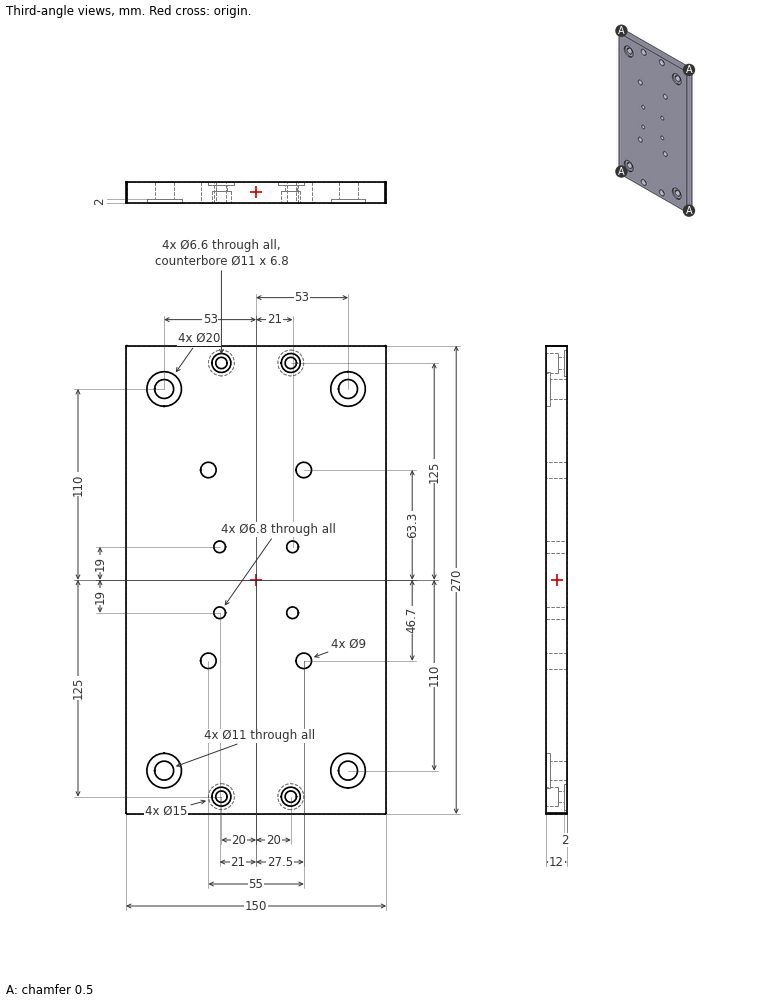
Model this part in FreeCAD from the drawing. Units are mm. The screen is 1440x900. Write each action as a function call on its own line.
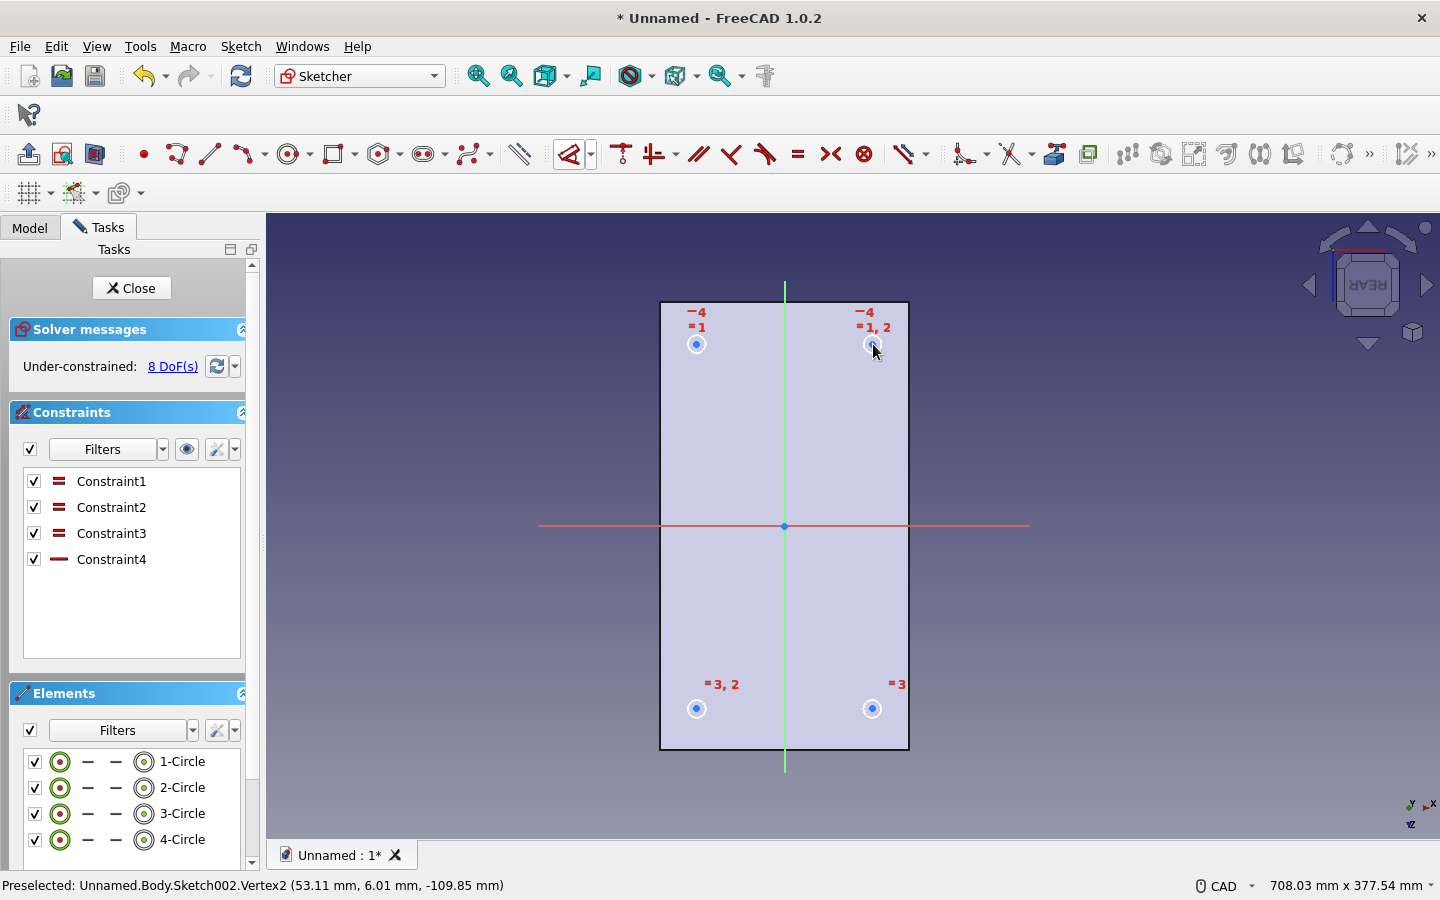
click(697, 344)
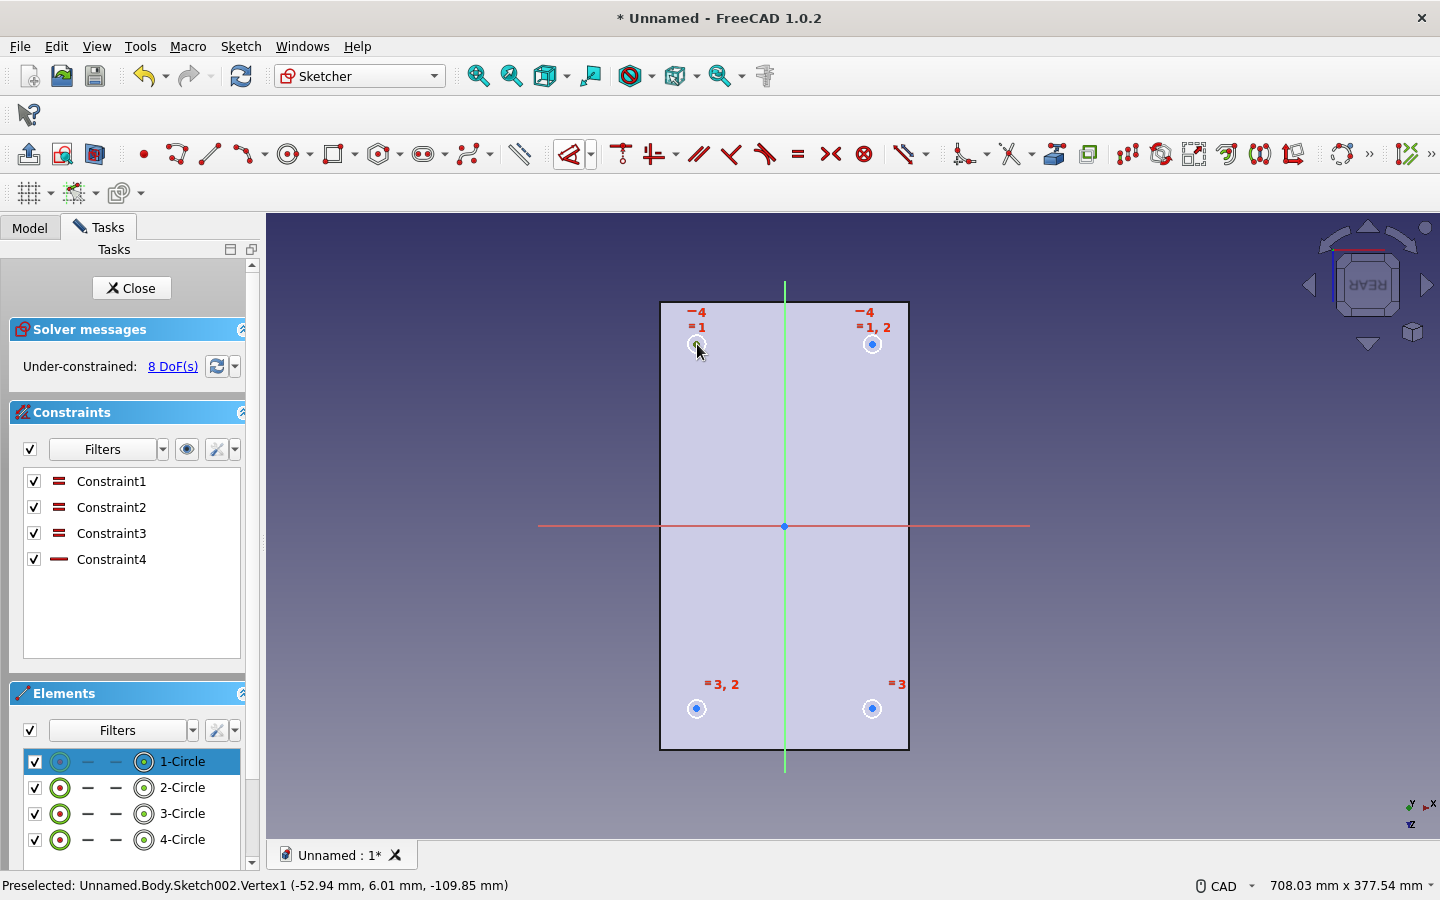
click(697, 709)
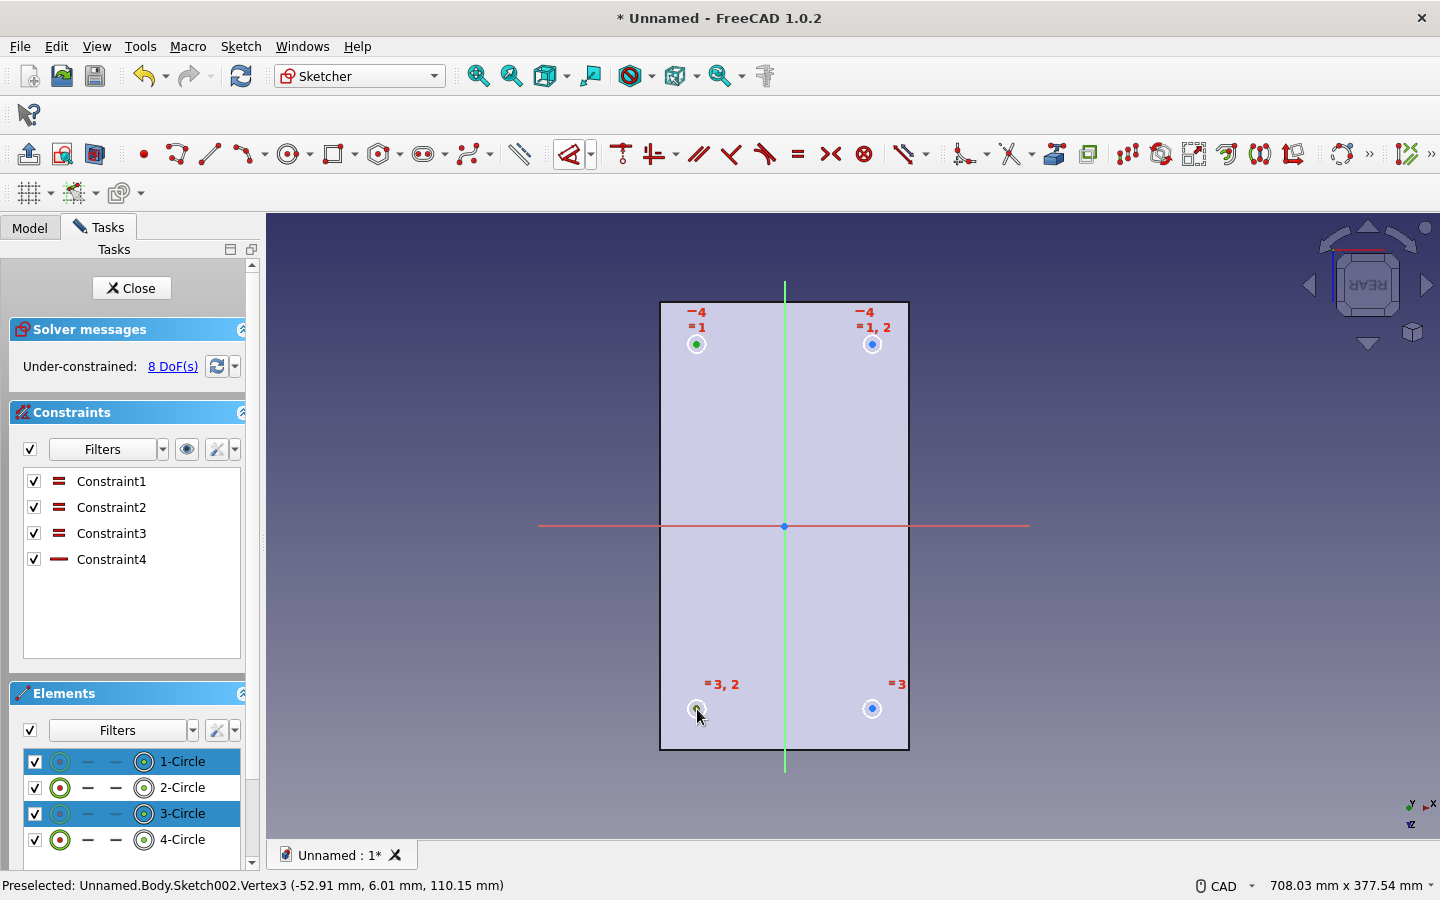
key(v)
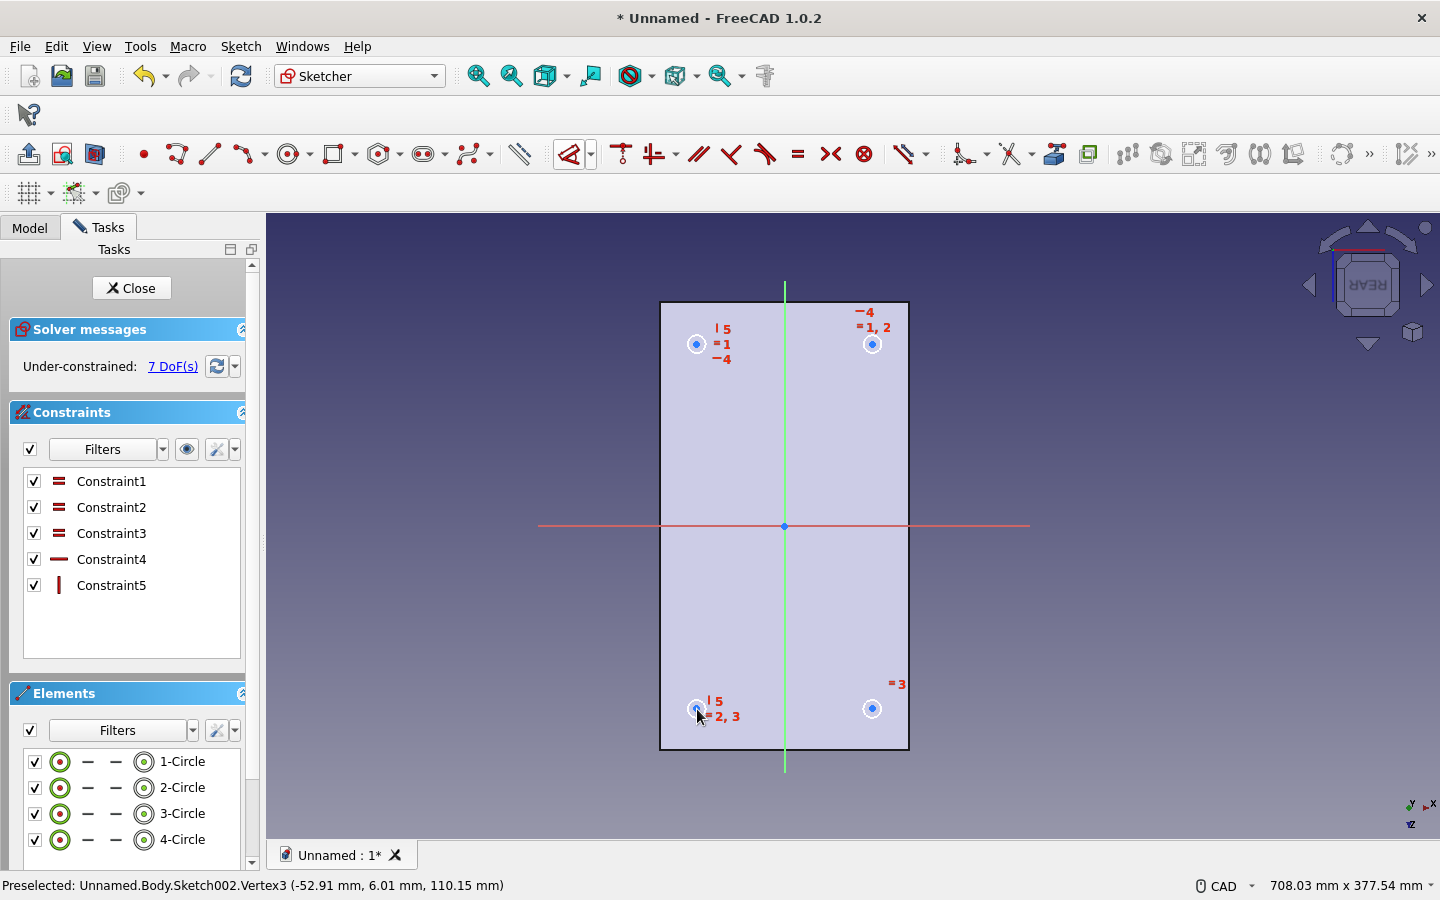
click(873, 344)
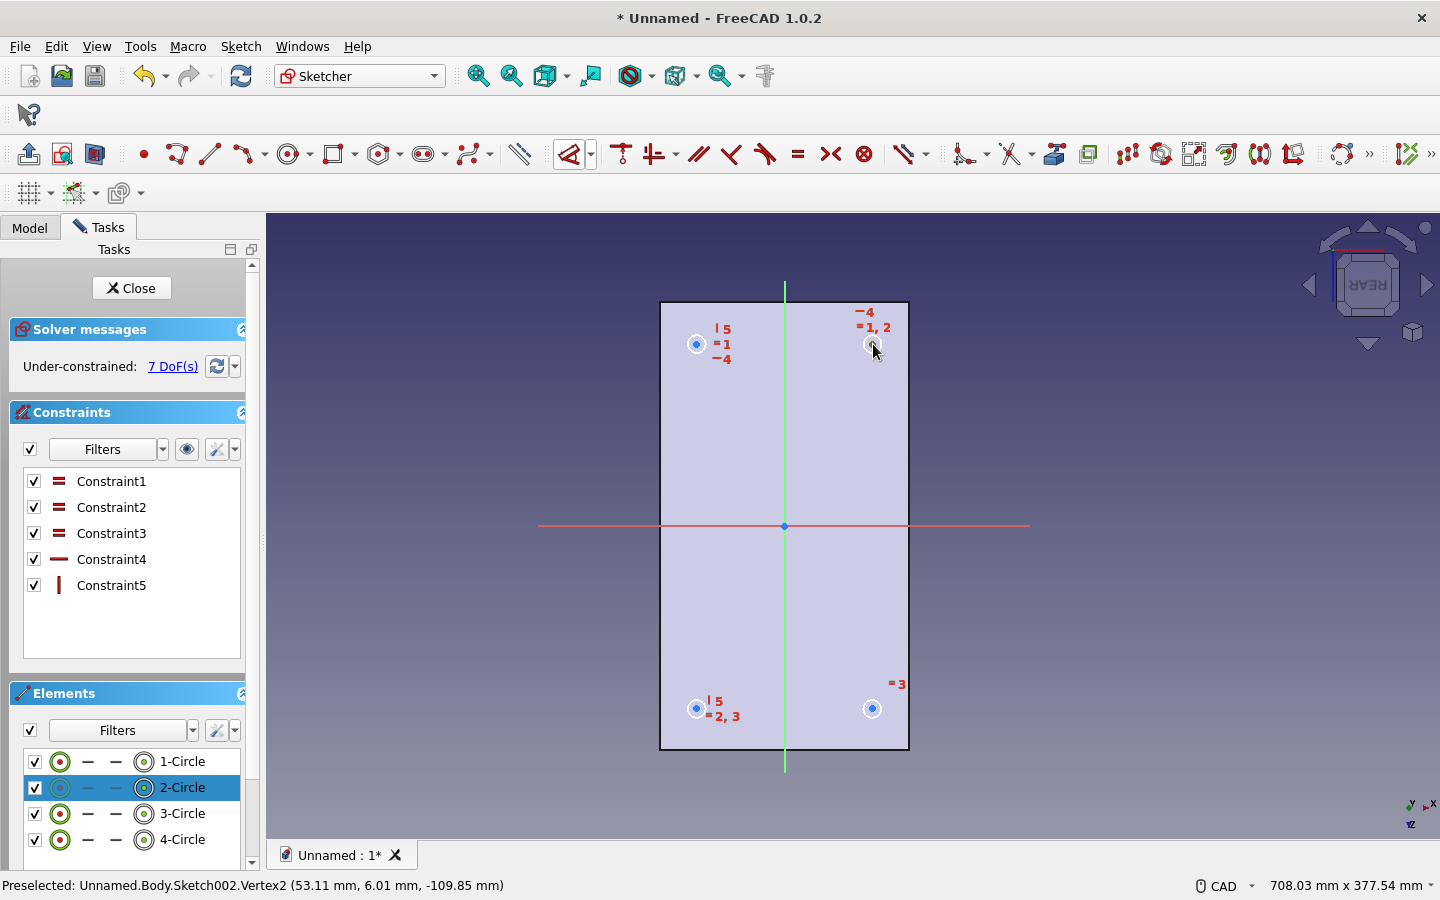
click(872, 709)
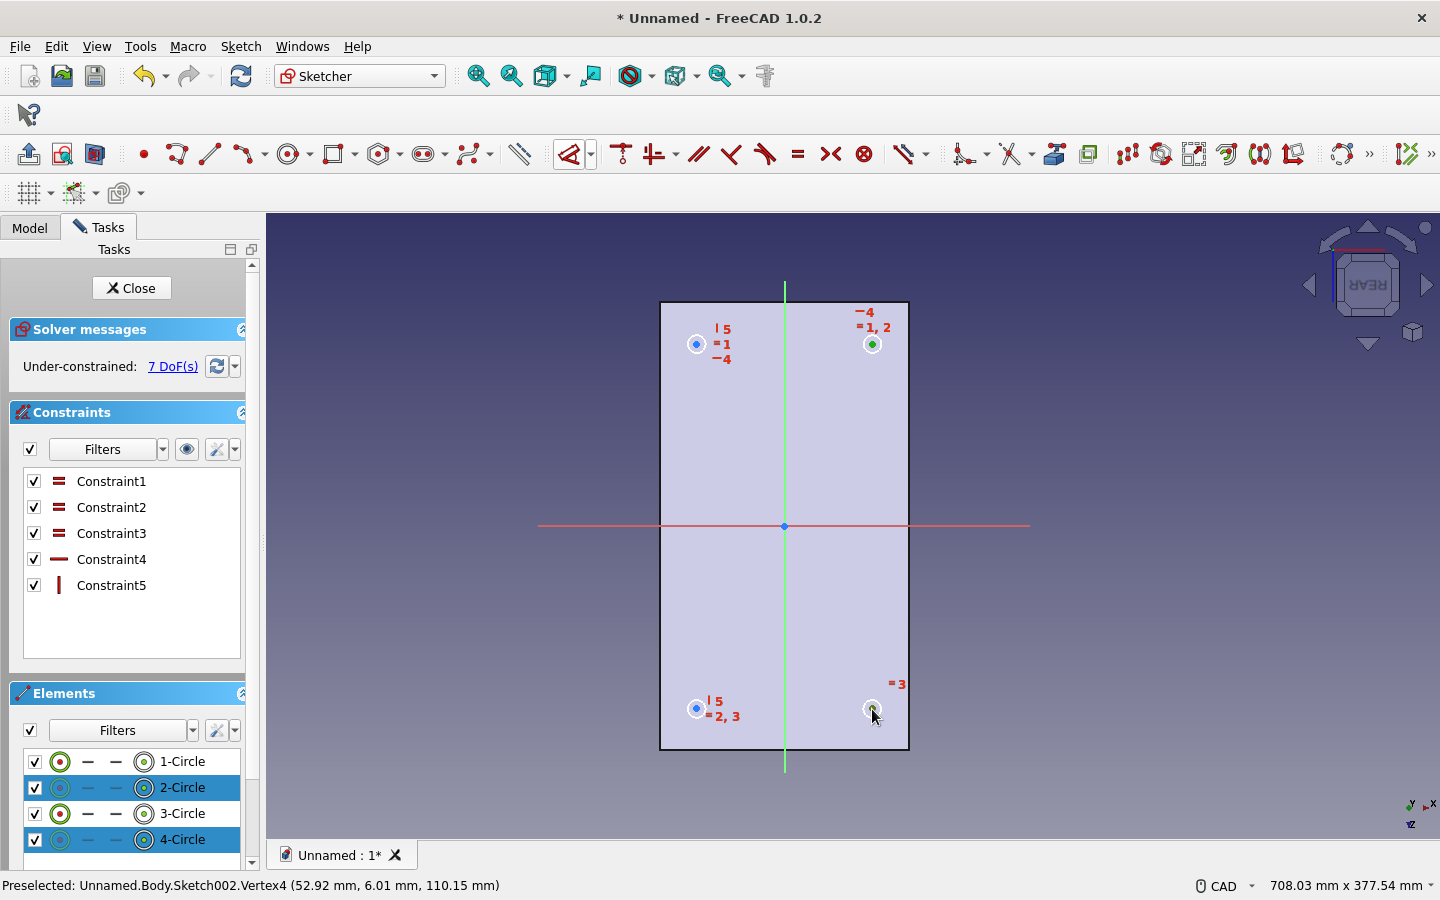
key(v)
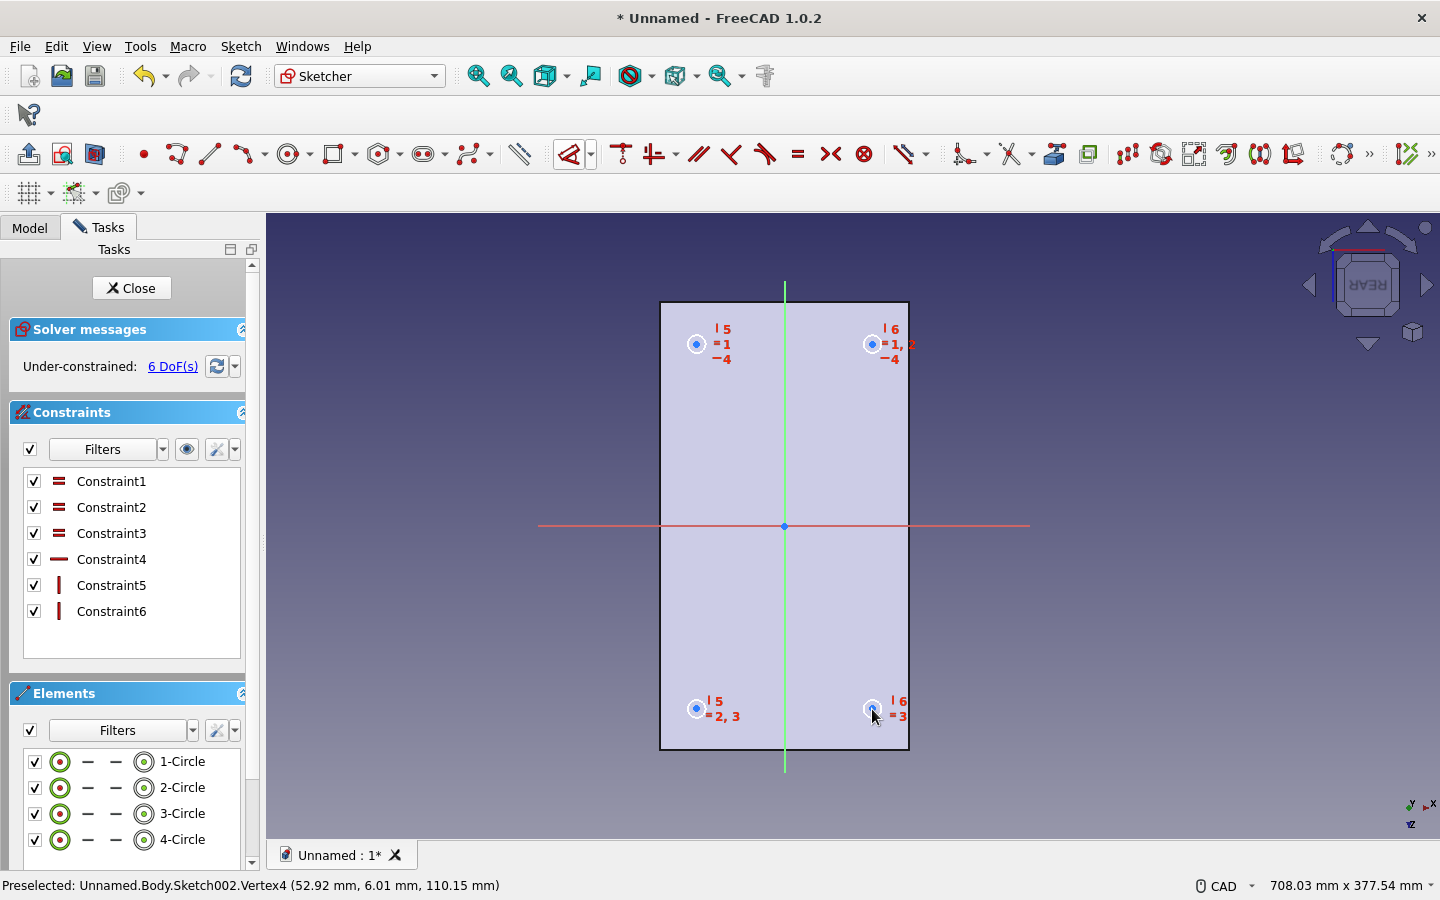
click(697, 709)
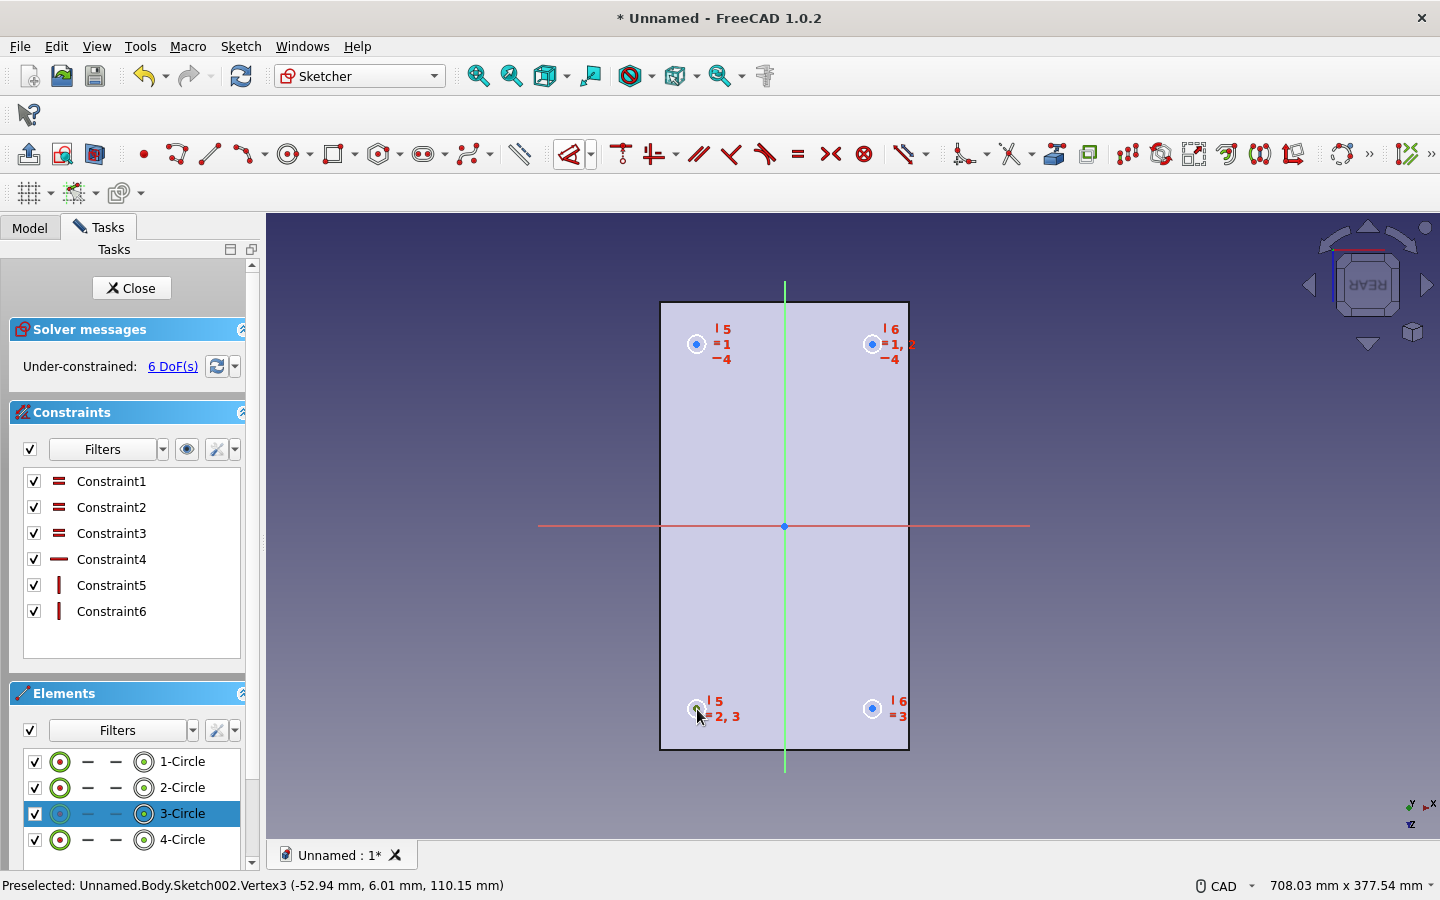
click(873, 709)